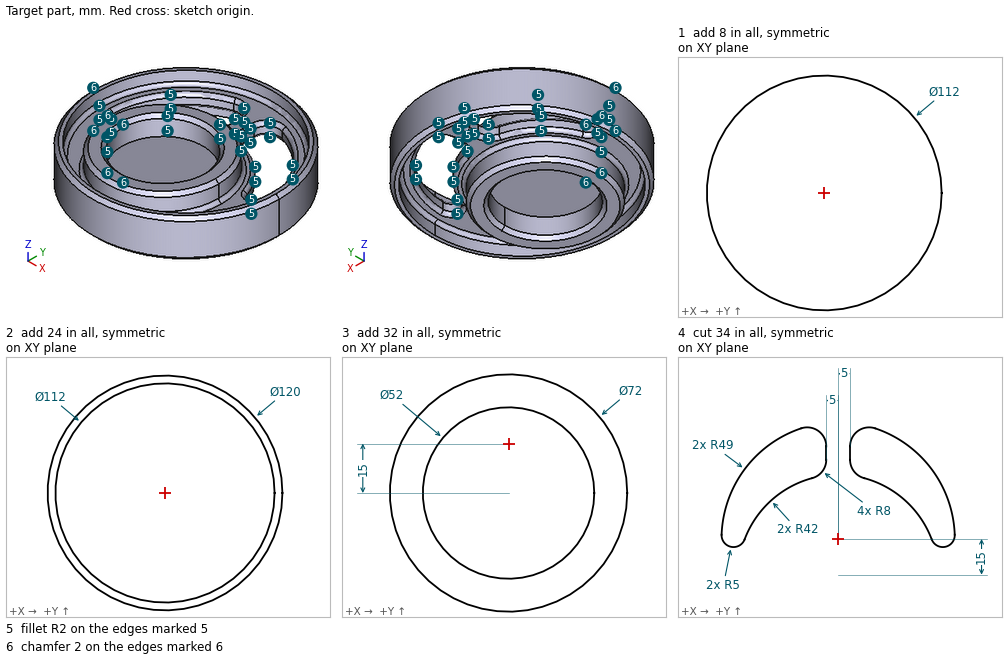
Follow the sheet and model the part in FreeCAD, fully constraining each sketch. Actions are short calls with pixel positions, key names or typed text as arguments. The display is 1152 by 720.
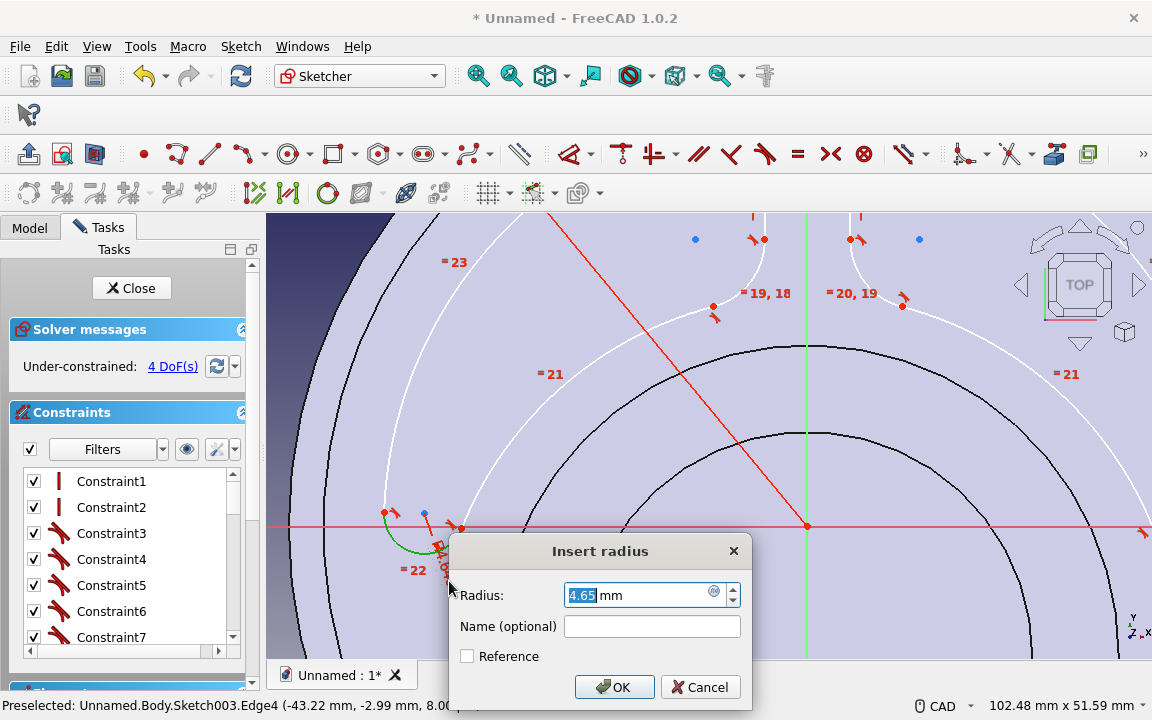
text(5)
key(Return)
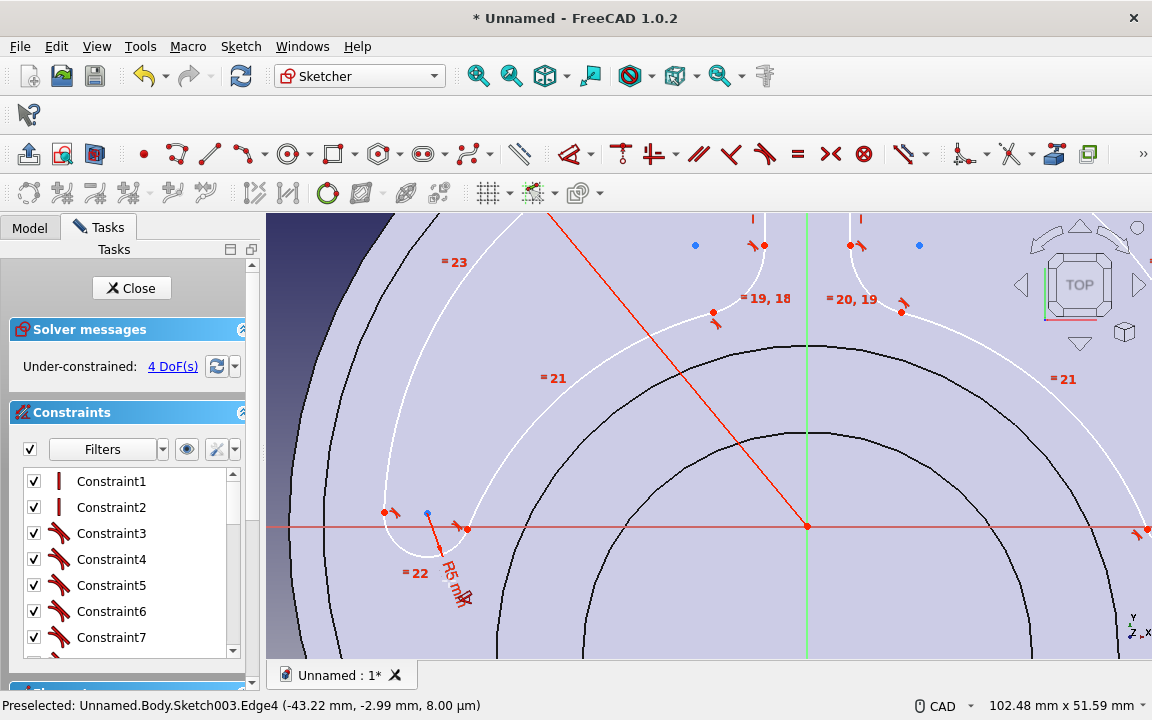
click(620, 352)
click(604, 324)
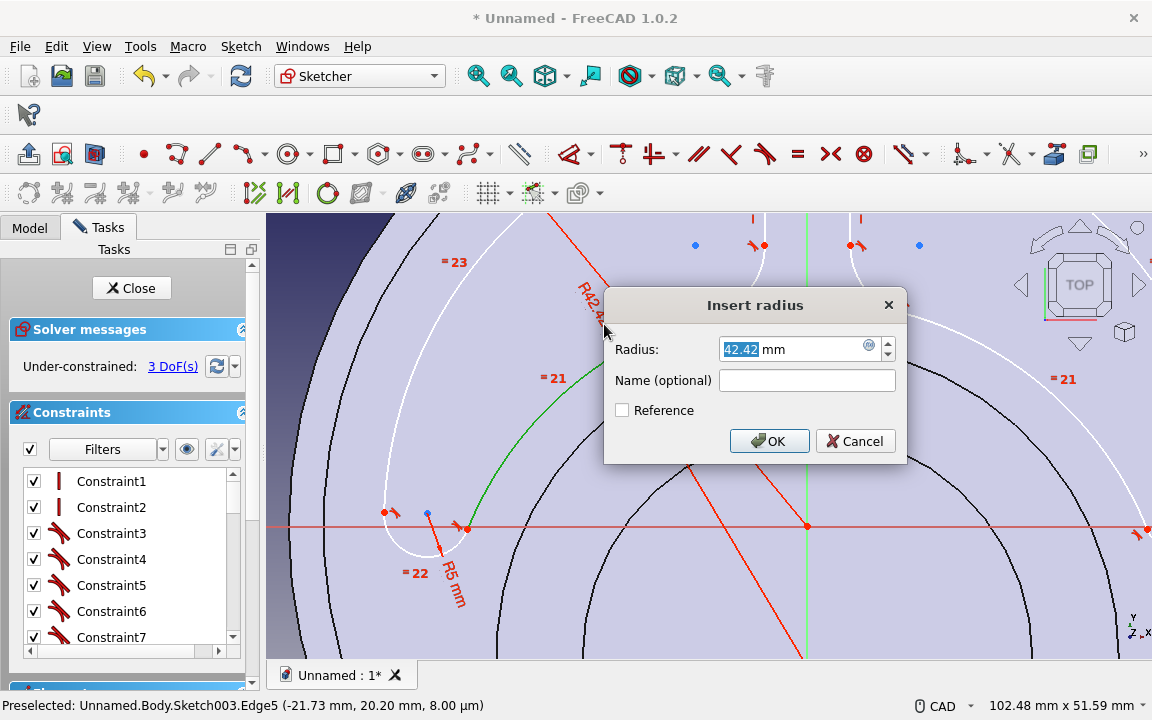
text(42)
key(Return)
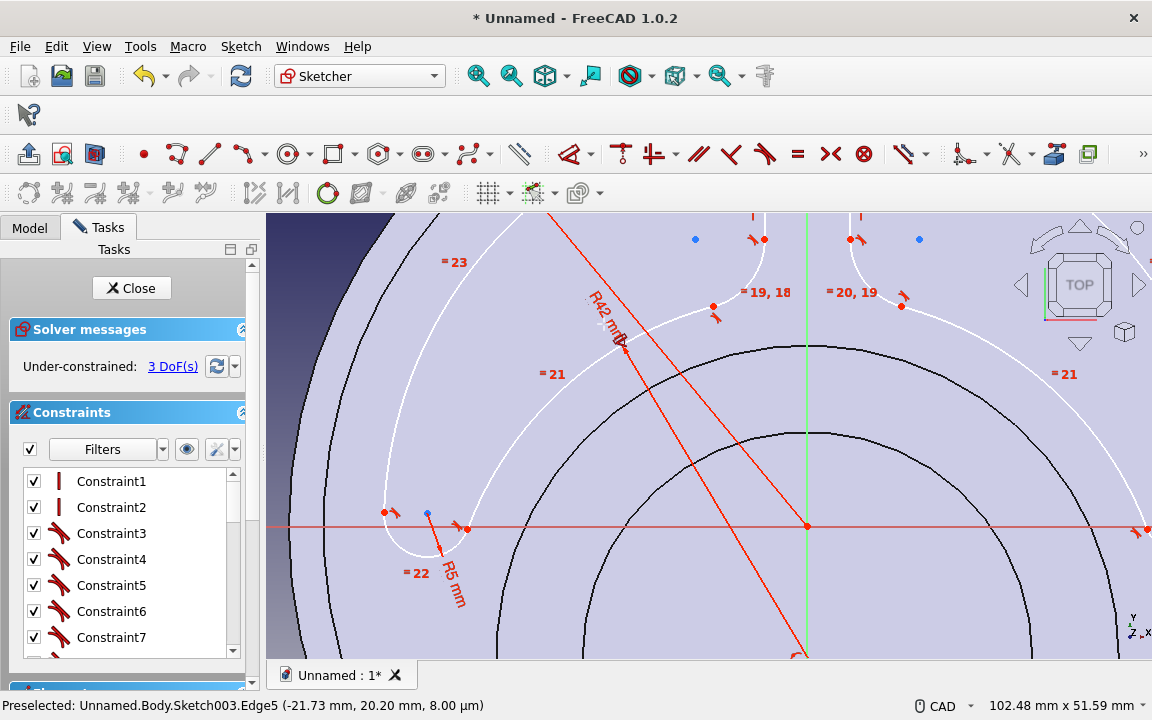
scroll(437, 552, down, 3)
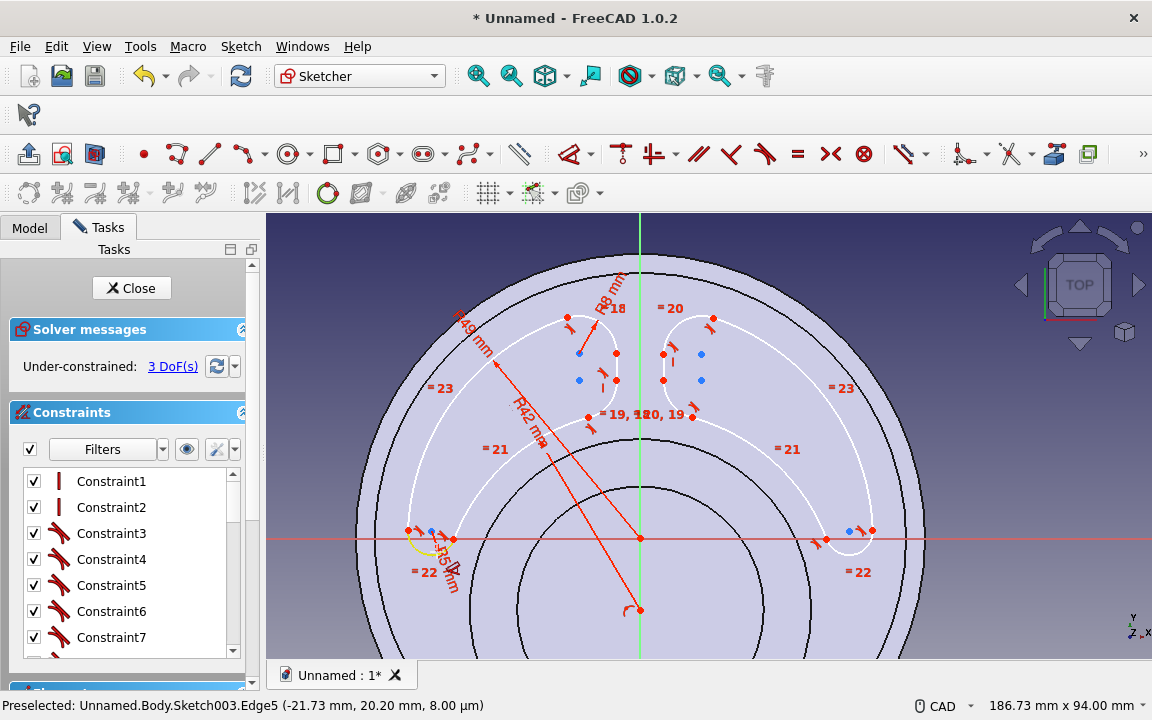
scroll(617, 381, up, 3)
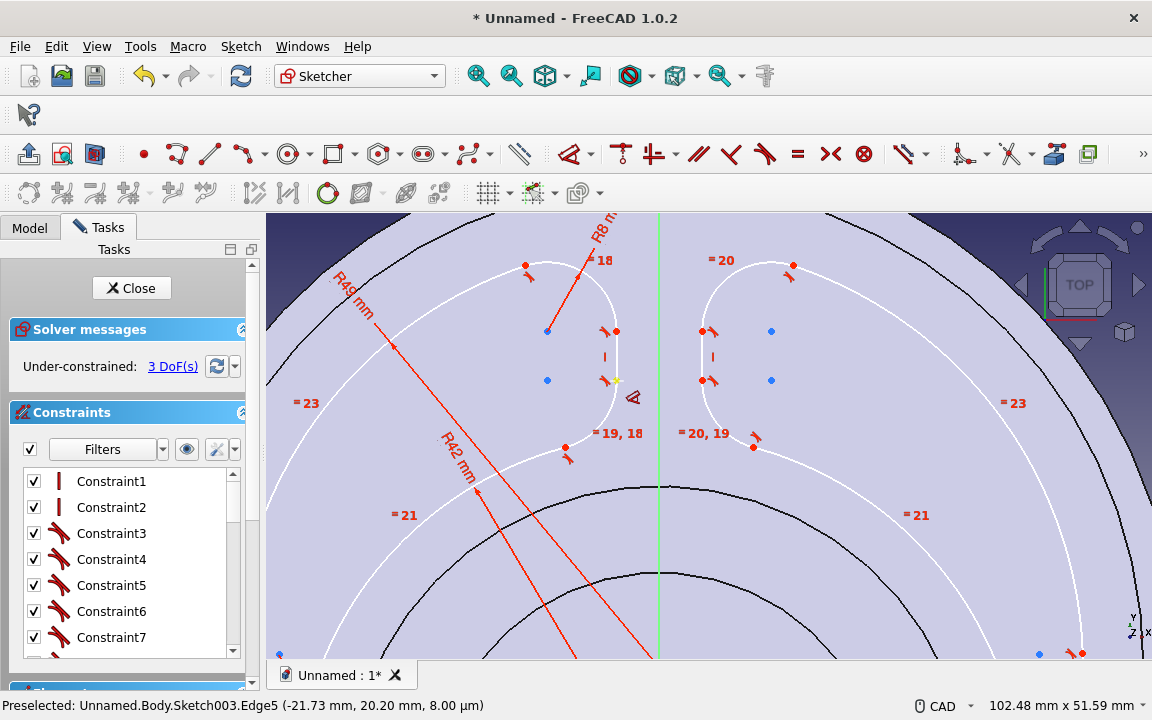
click(617, 381)
click(638, 347)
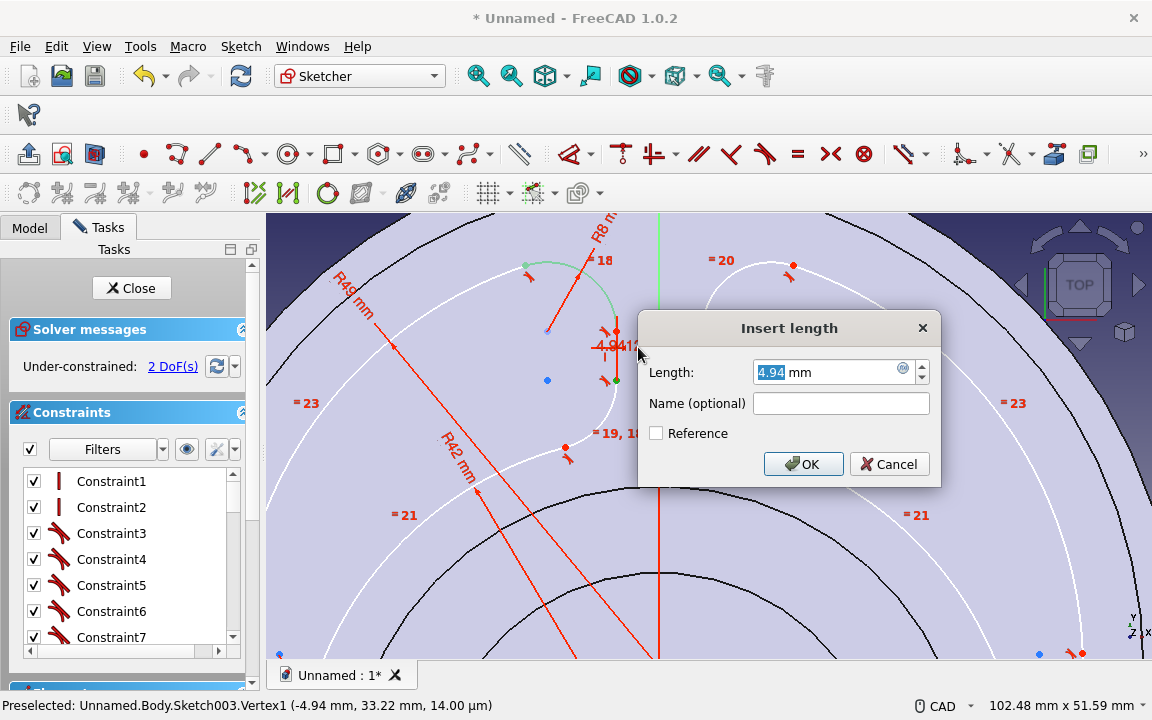
text(5)
key(Return)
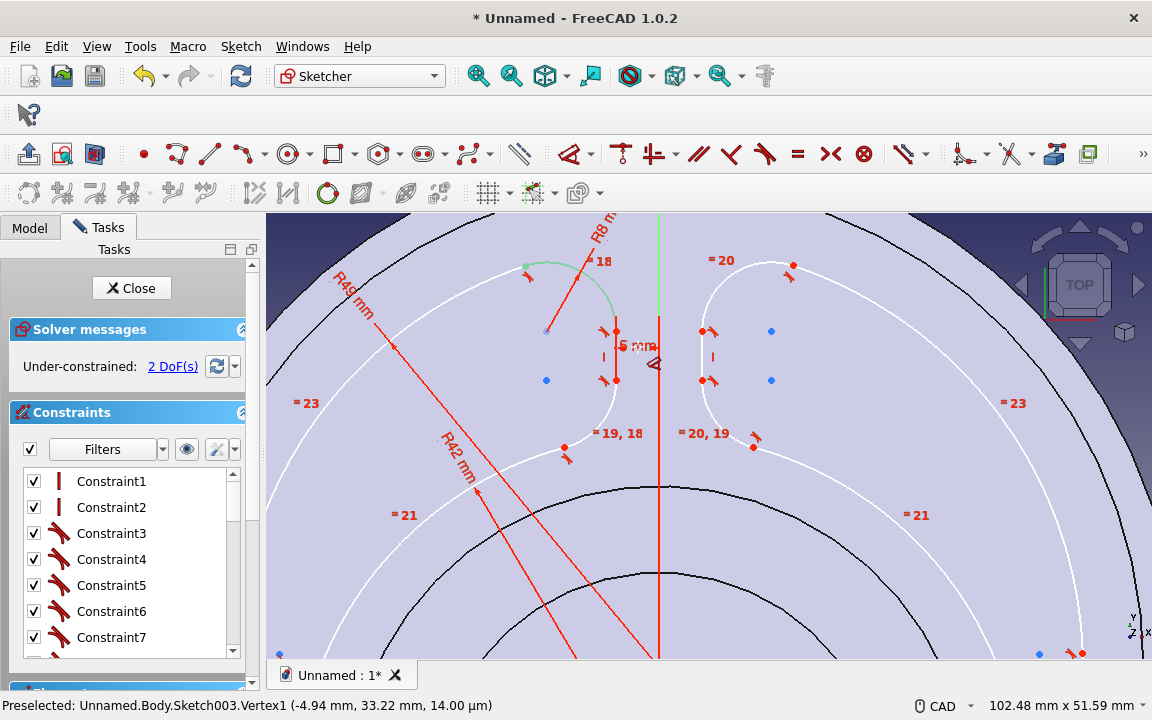
click(702, 332)
click(681, 298)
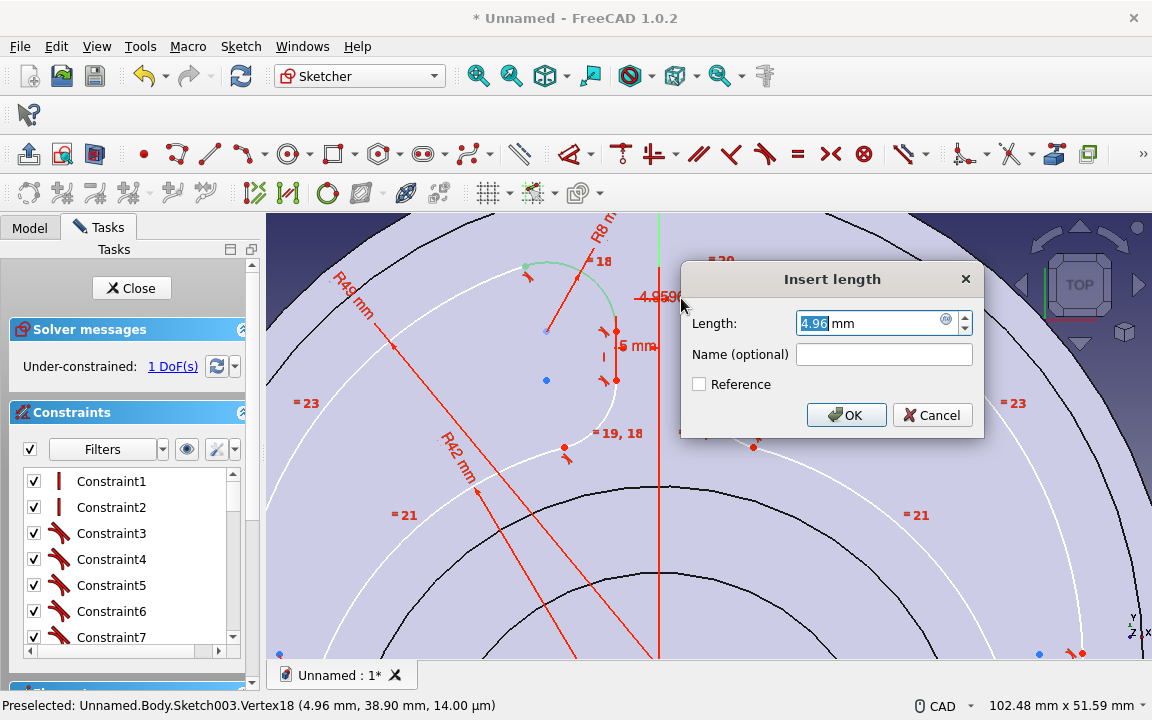
text(5)
key(Return)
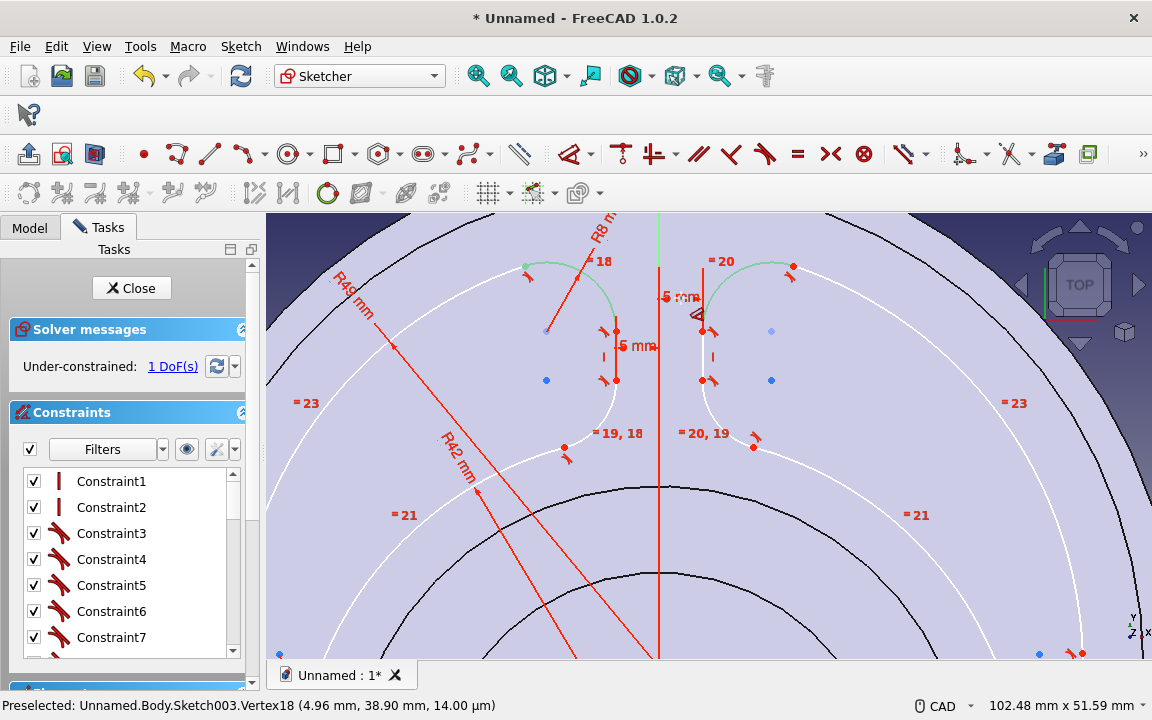
scroll(618, 381, down, 3)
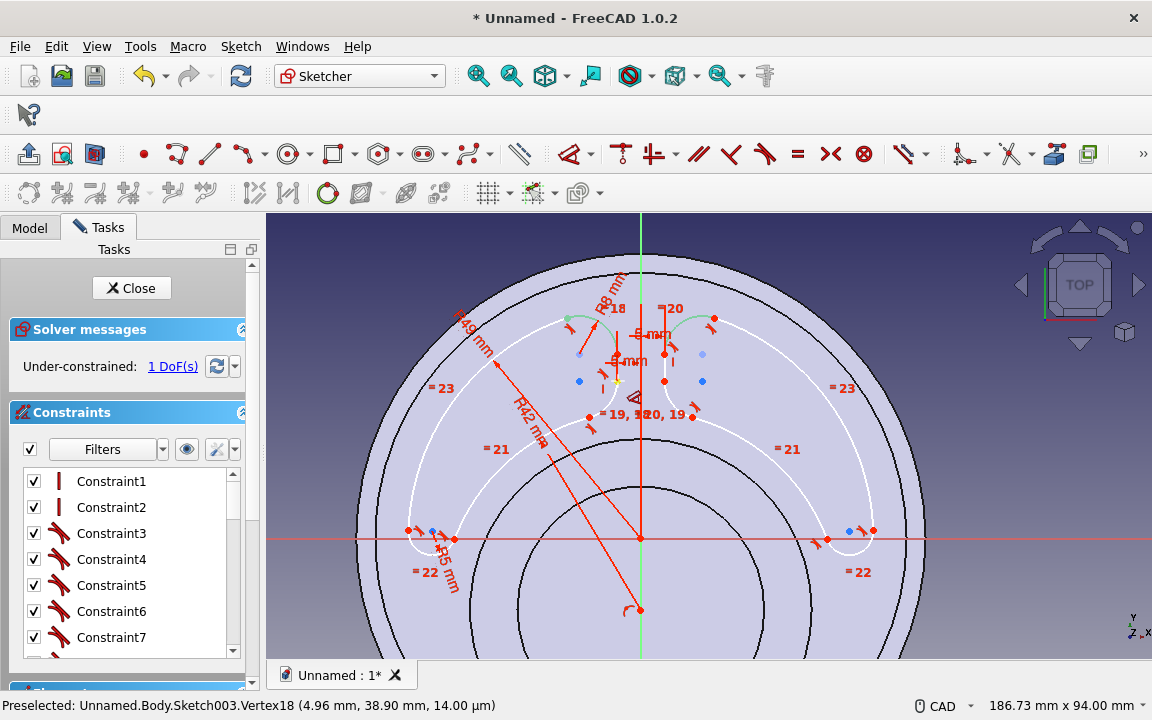
click(641, 610)
click(675, 574)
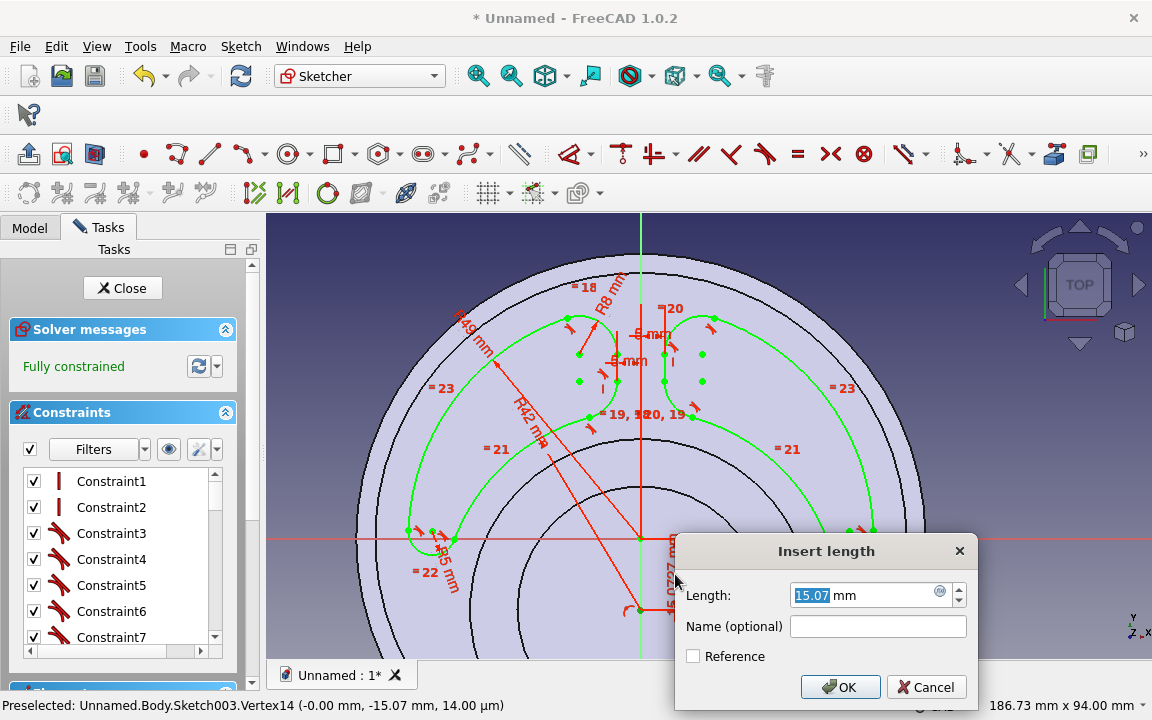
text(15)
key(Return)
key(Escape)